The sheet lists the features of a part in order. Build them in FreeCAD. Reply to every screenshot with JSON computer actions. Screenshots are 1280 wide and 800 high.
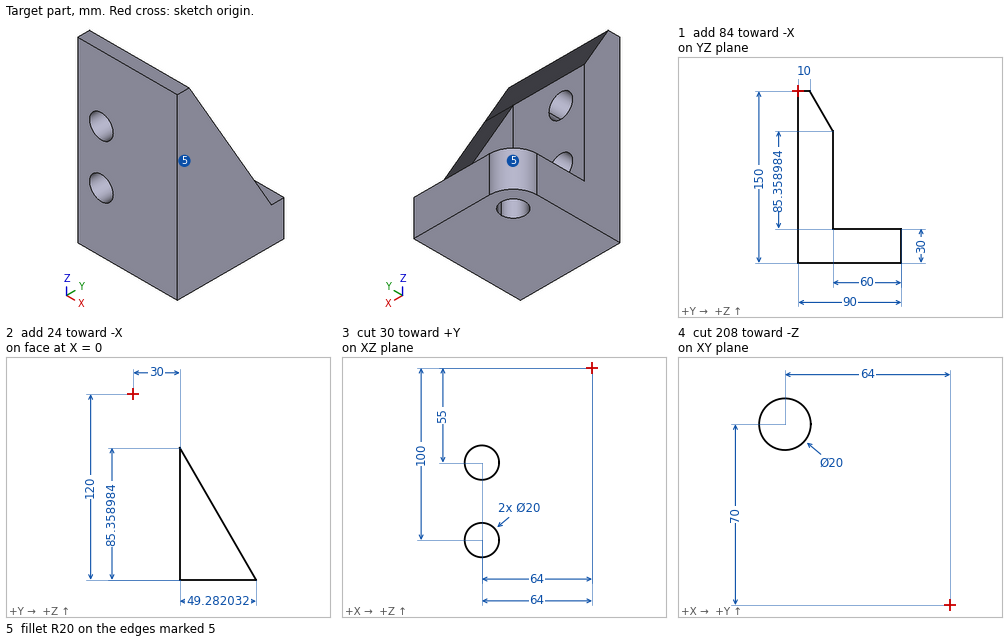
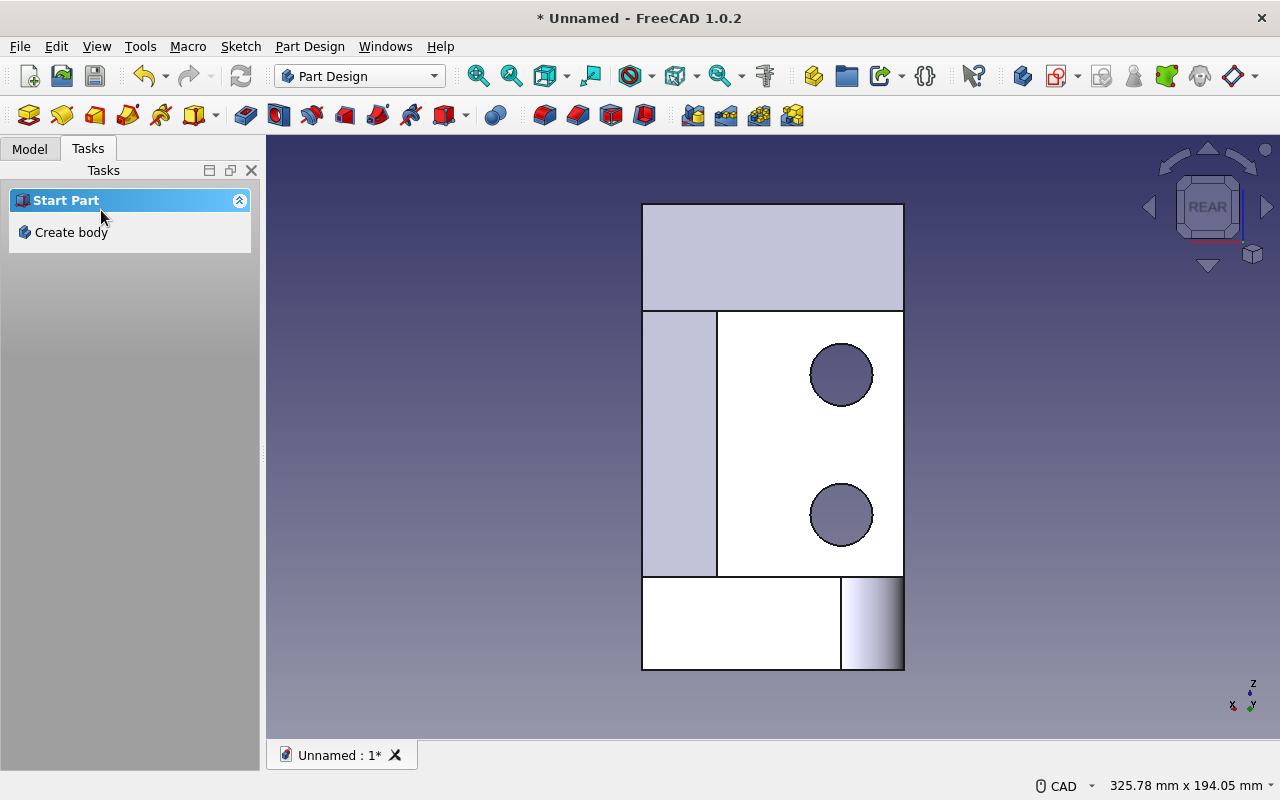
{"action": "key", "text": "0"}